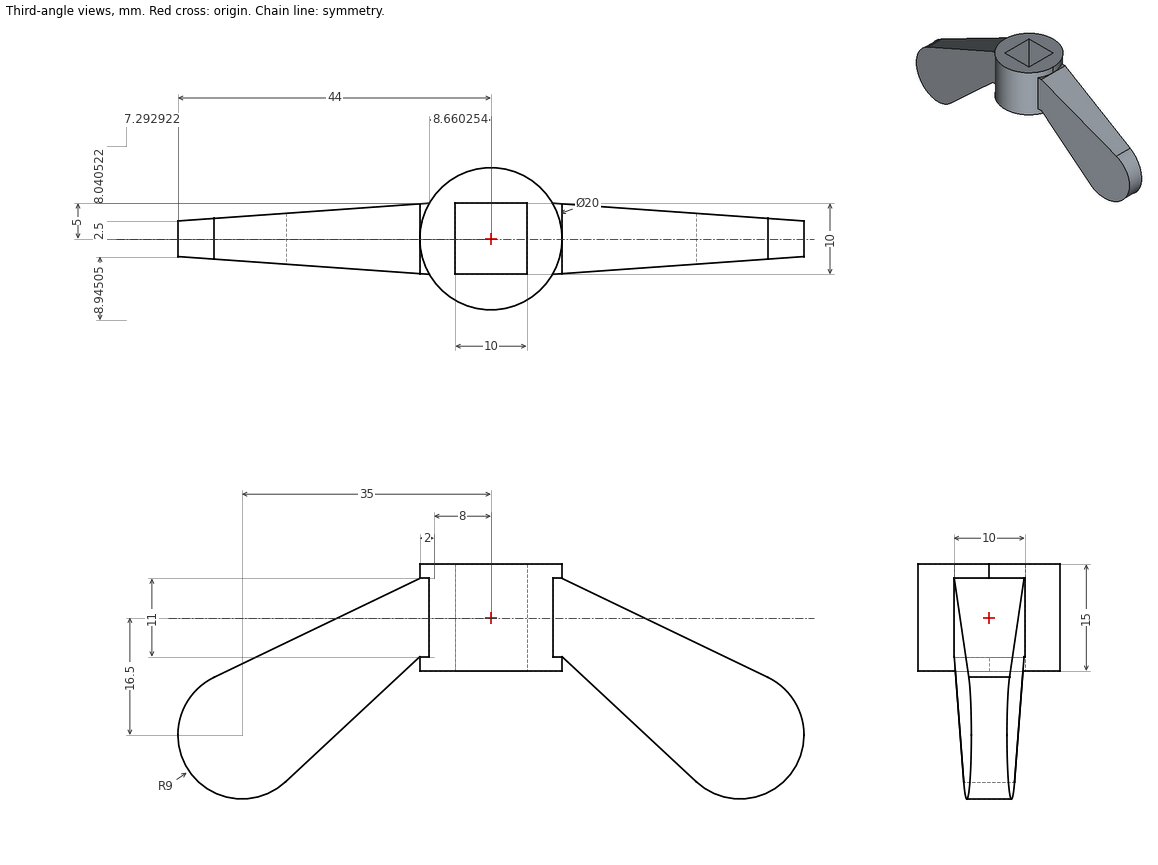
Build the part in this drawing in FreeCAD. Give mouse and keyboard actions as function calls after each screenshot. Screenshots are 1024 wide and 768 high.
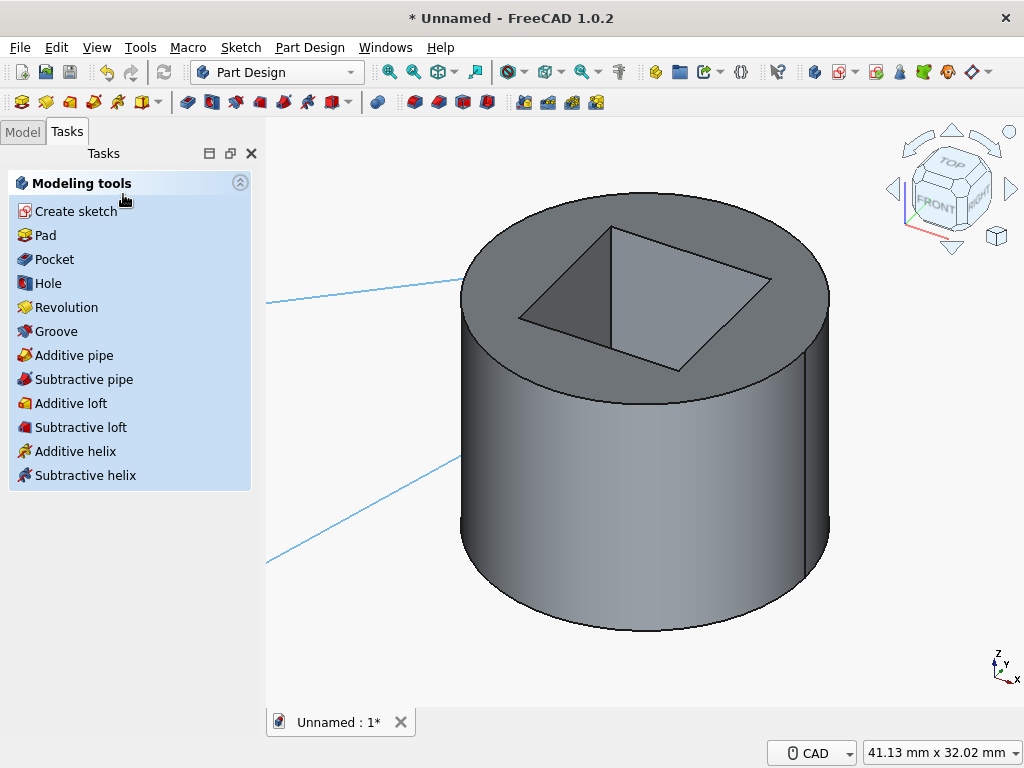
click(22, 102)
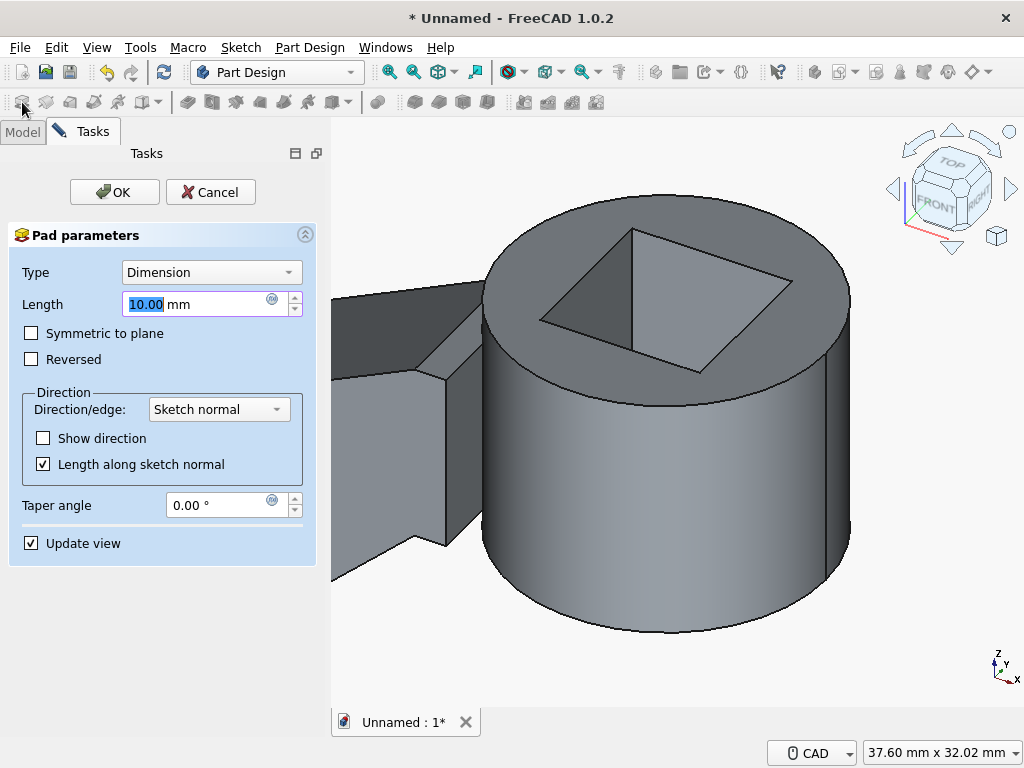
text(10)
key(Tab)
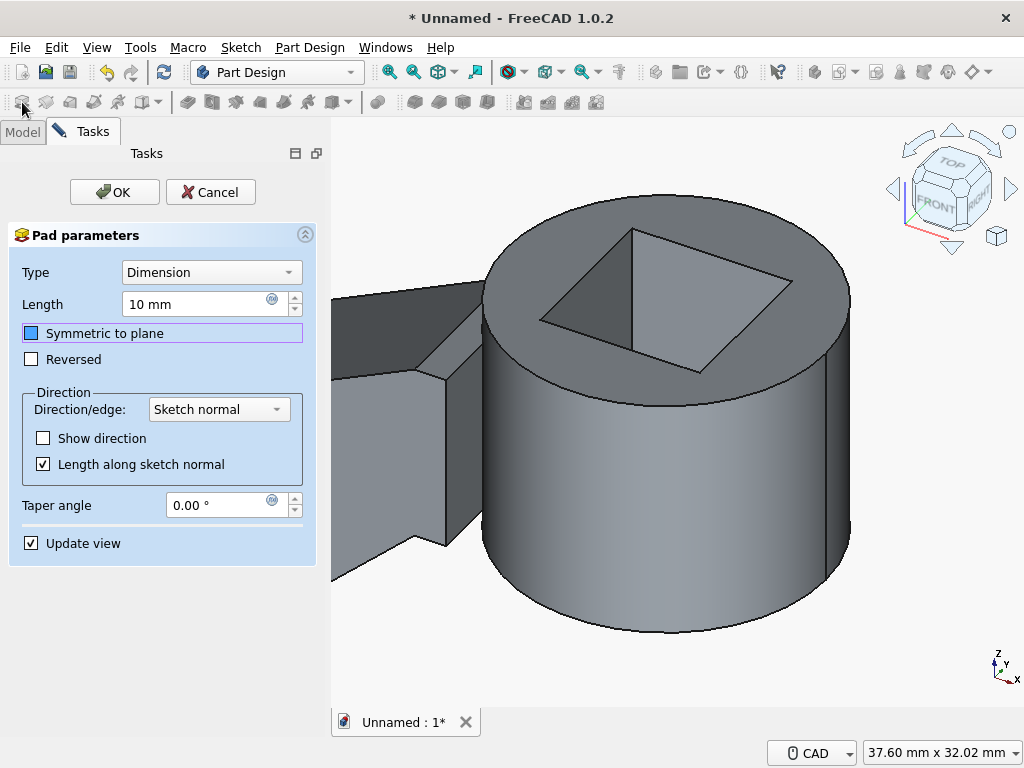
click(30, 333)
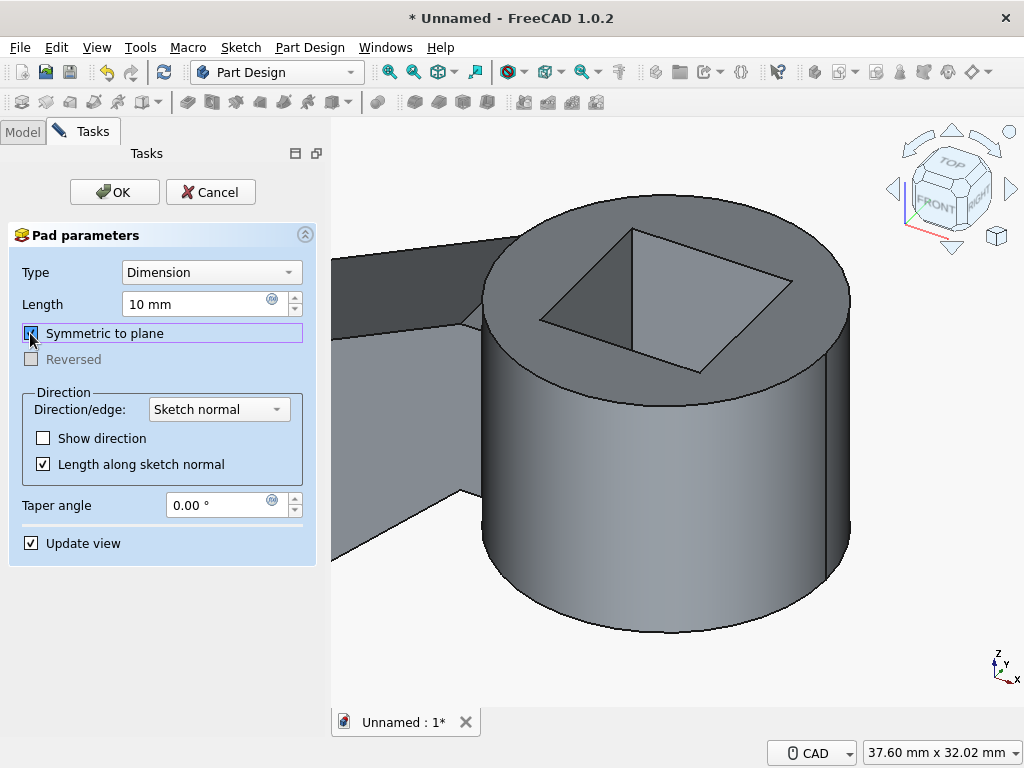
click(115, 192)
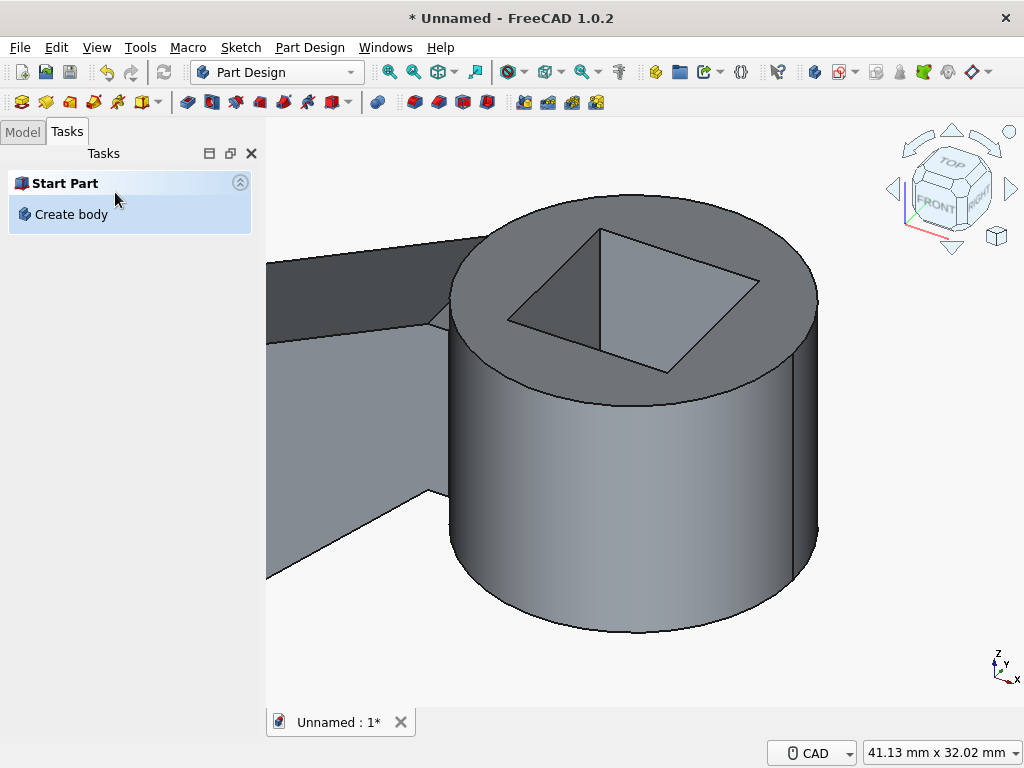
key(v)
key(f)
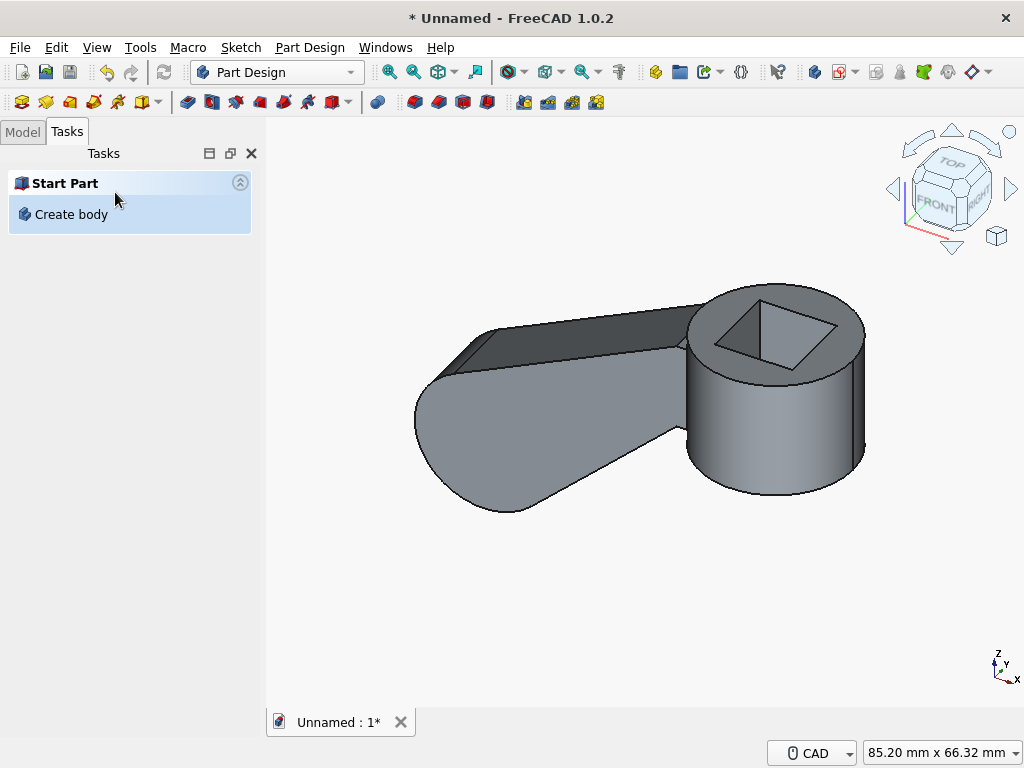
click(840, 72)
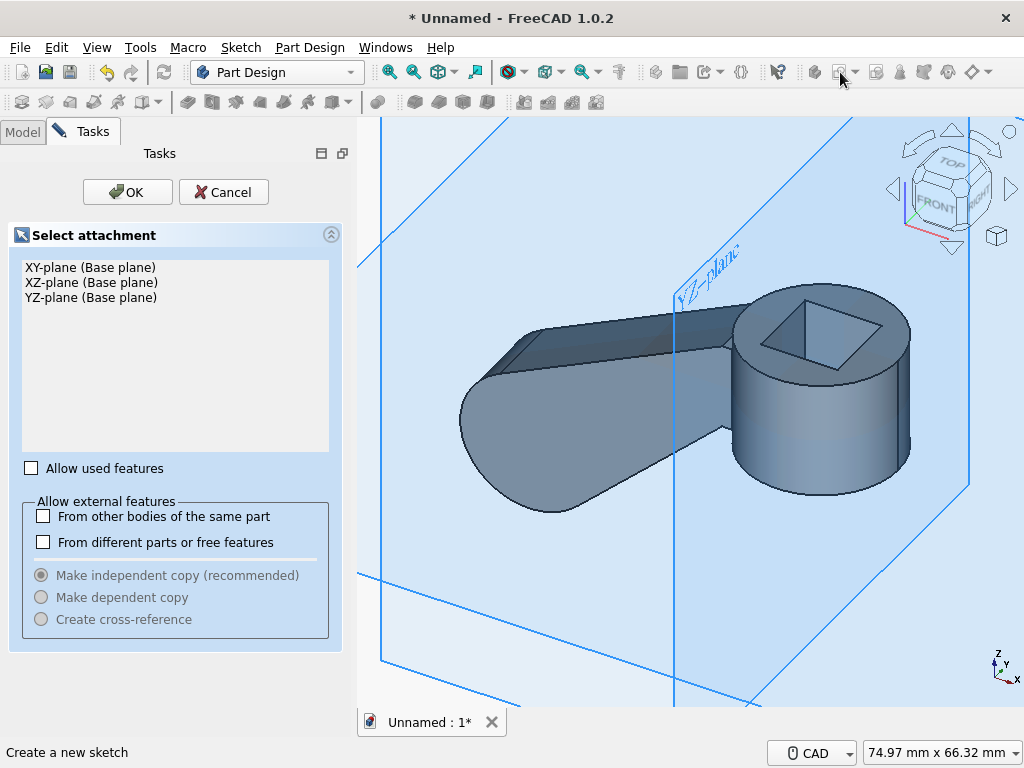
click(82, 268)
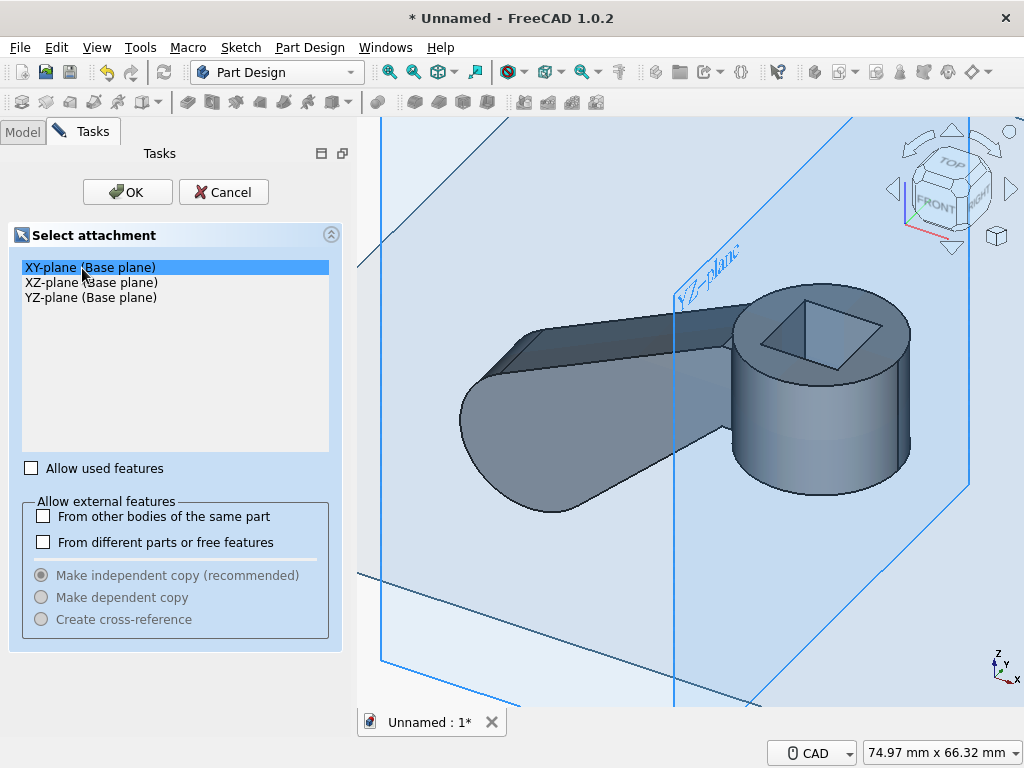
click(128, 192)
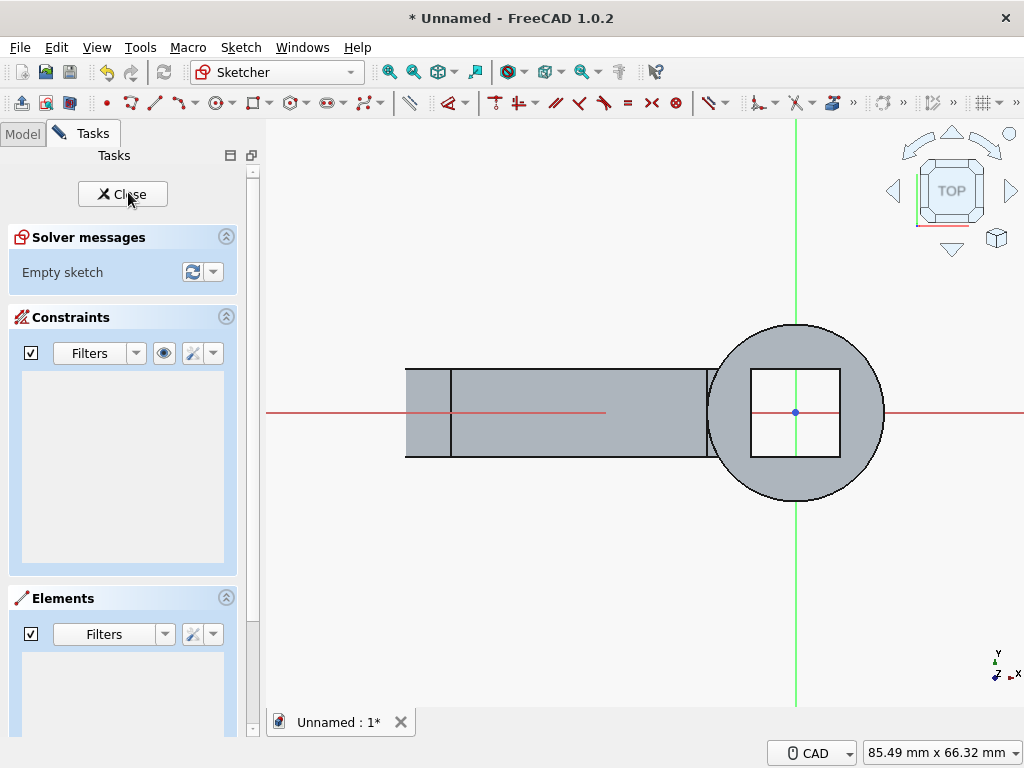
click(70, 104)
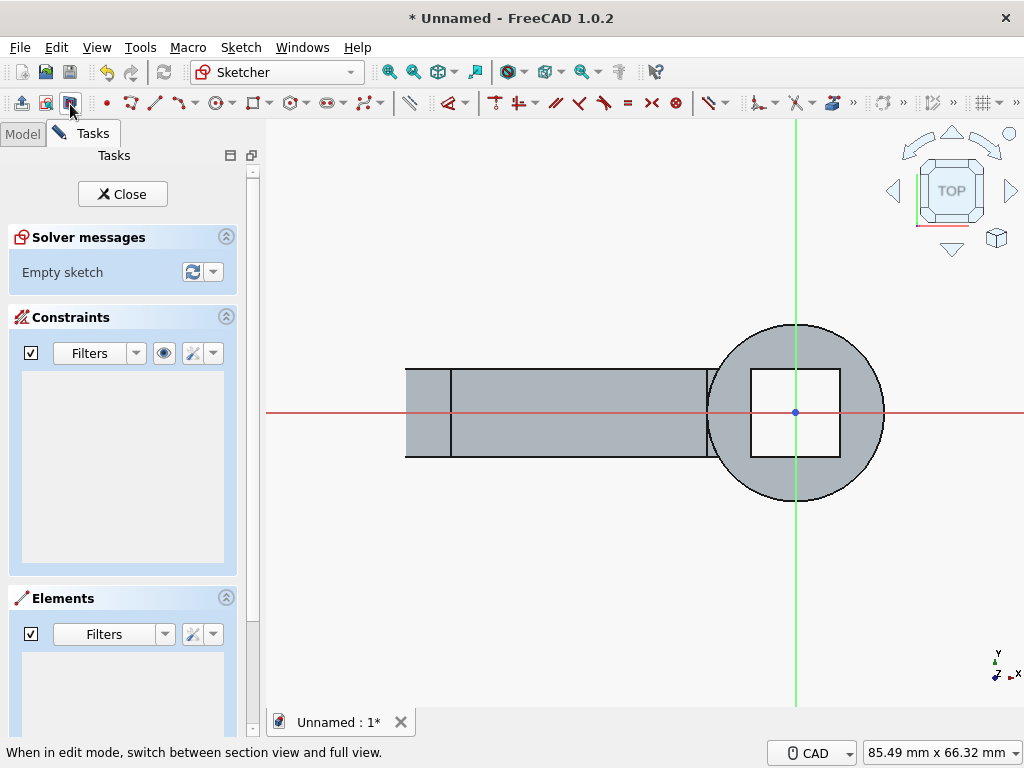
click(132, 104)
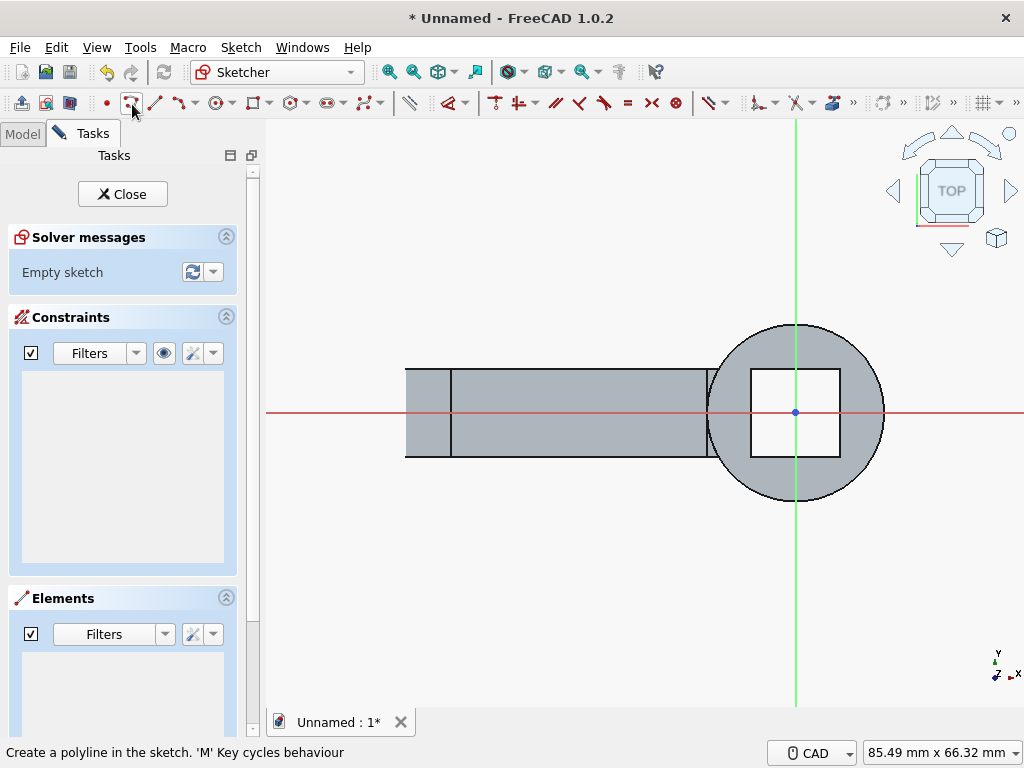
click(719, 369)
click(341, 297)
click(405, 391)
click(719, 370)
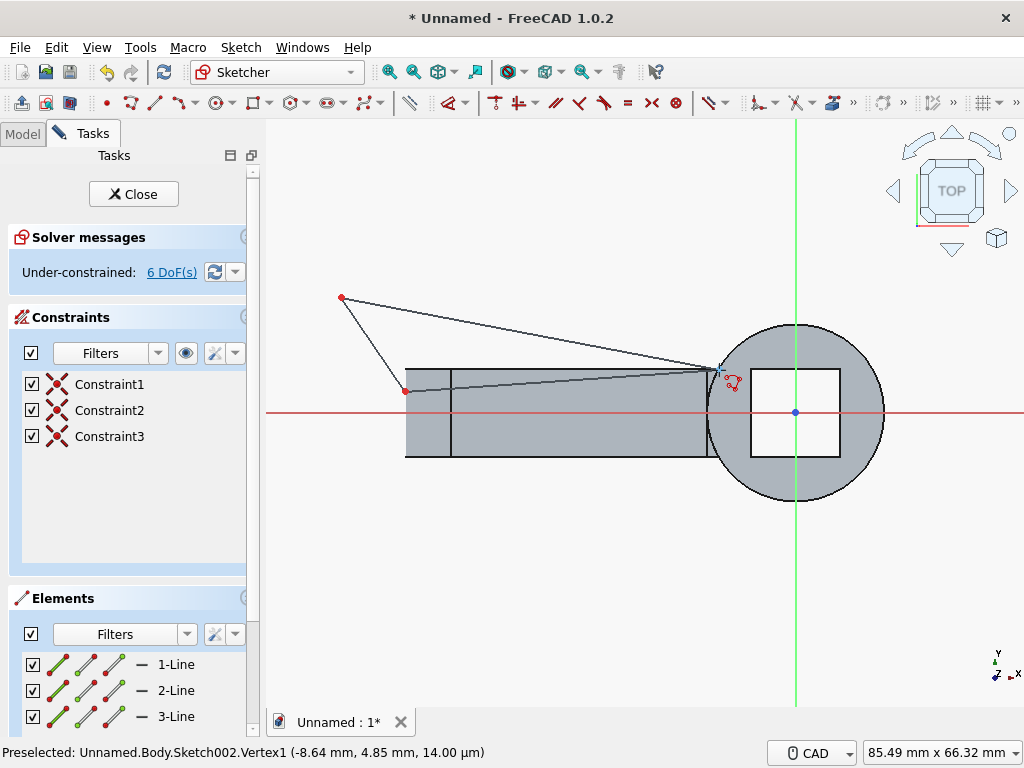
click(719, 457)
click(405, 435)
click(341, 514)
click(719, 458)
key(Escape)
key(Escape)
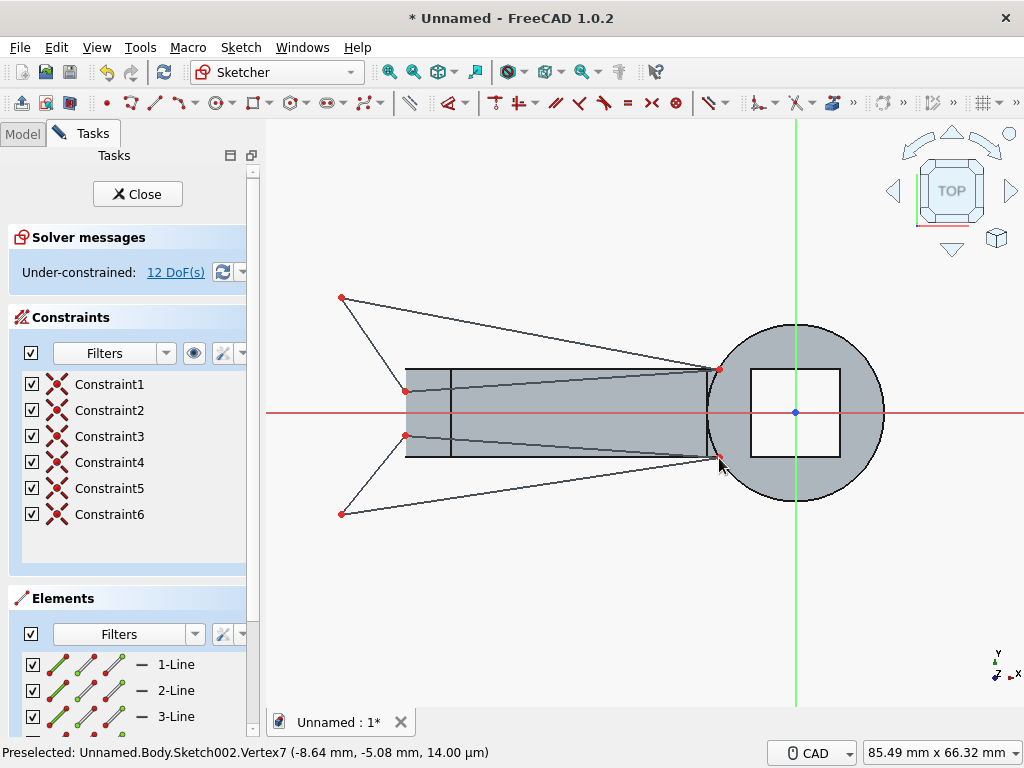
click(719, 370)